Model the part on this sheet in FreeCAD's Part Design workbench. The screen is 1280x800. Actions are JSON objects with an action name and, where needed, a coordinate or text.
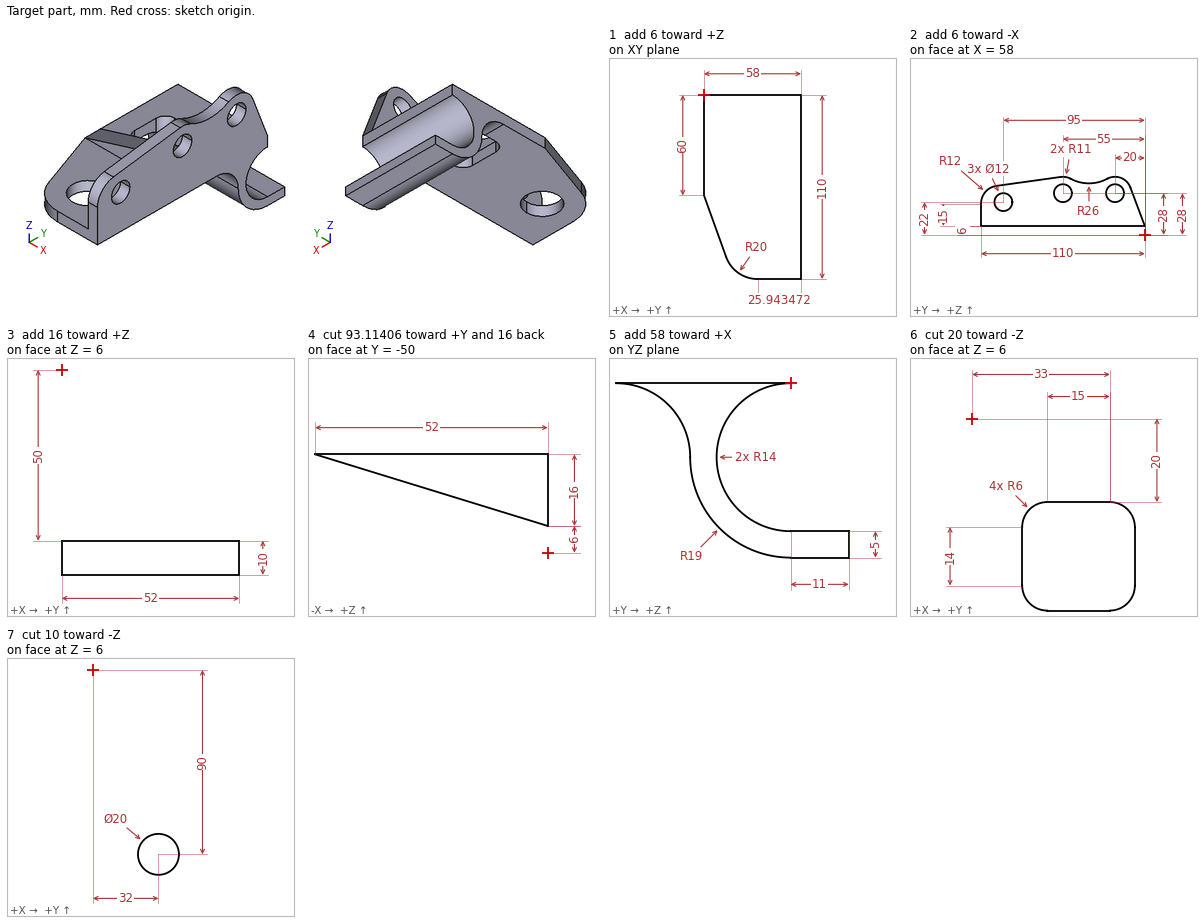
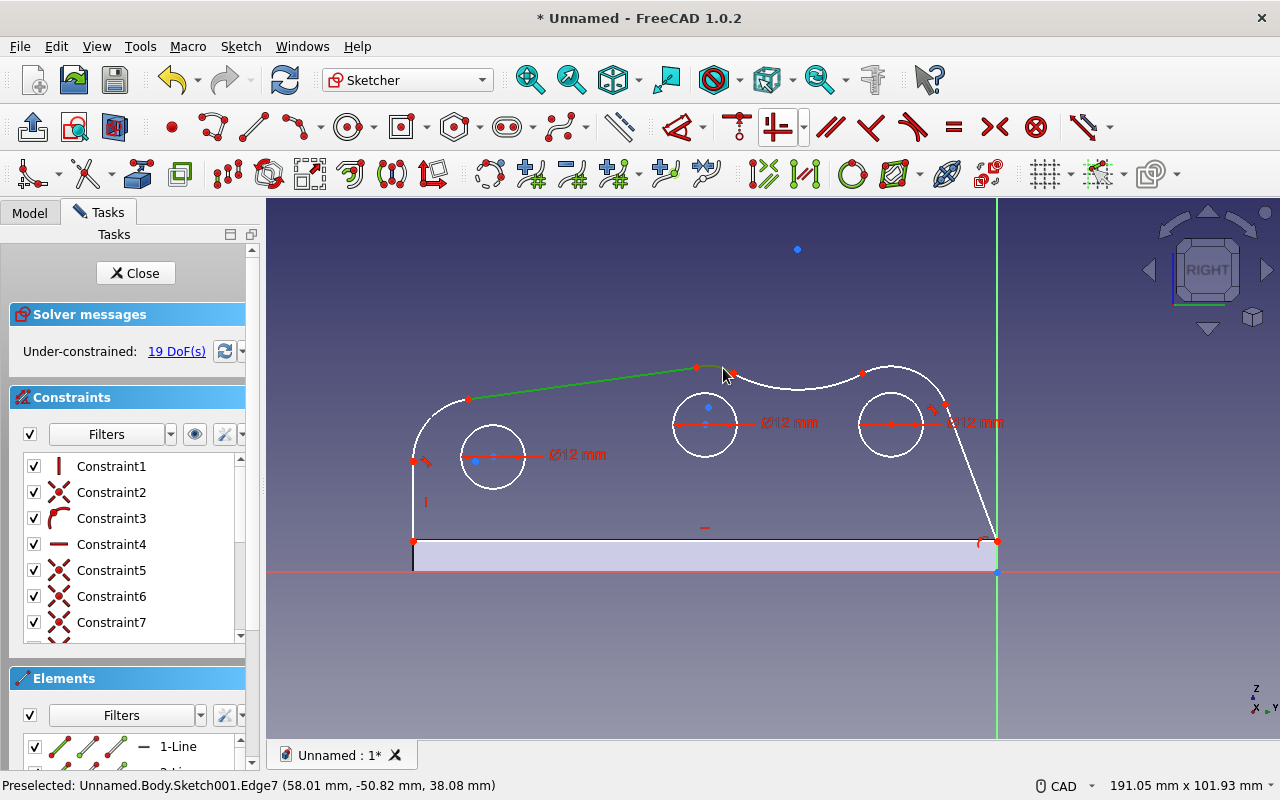
{"action": "key", "text": "t"}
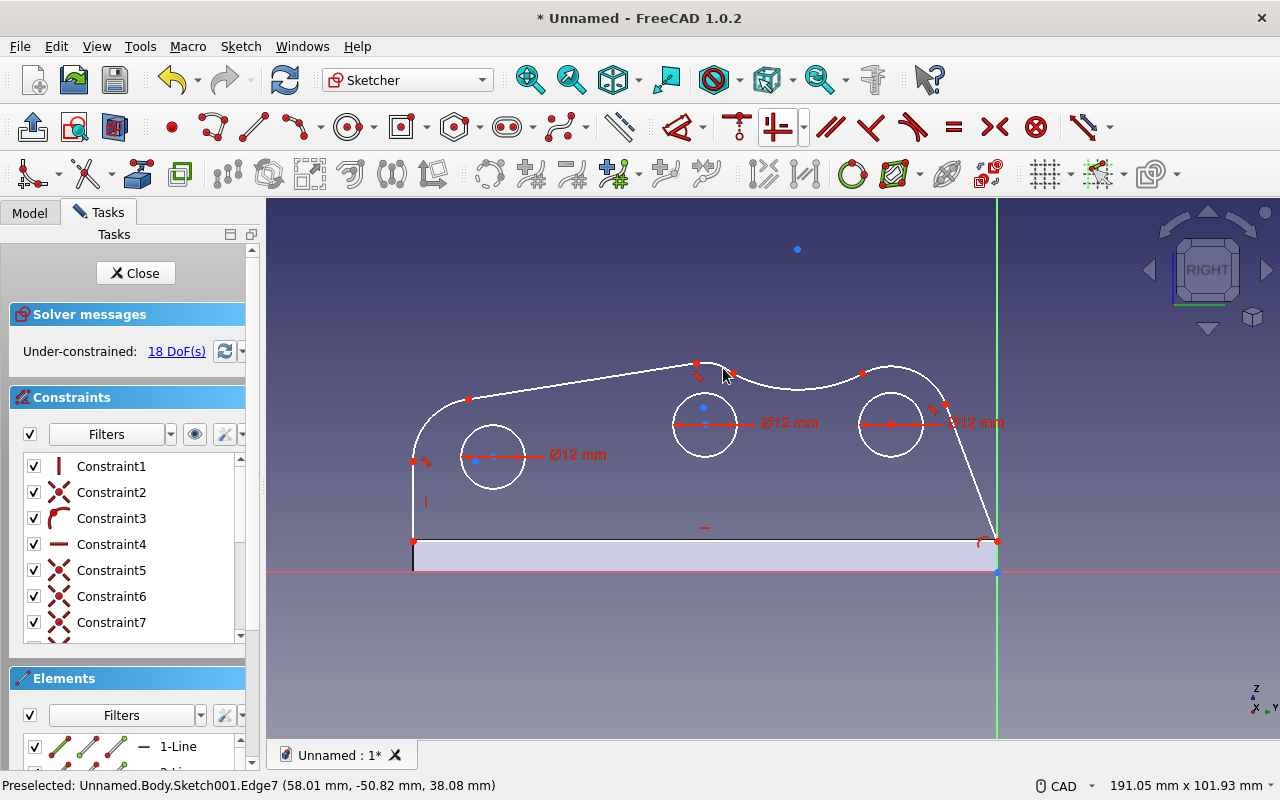
{"action": "left_click", "coordinate": [628, 374]}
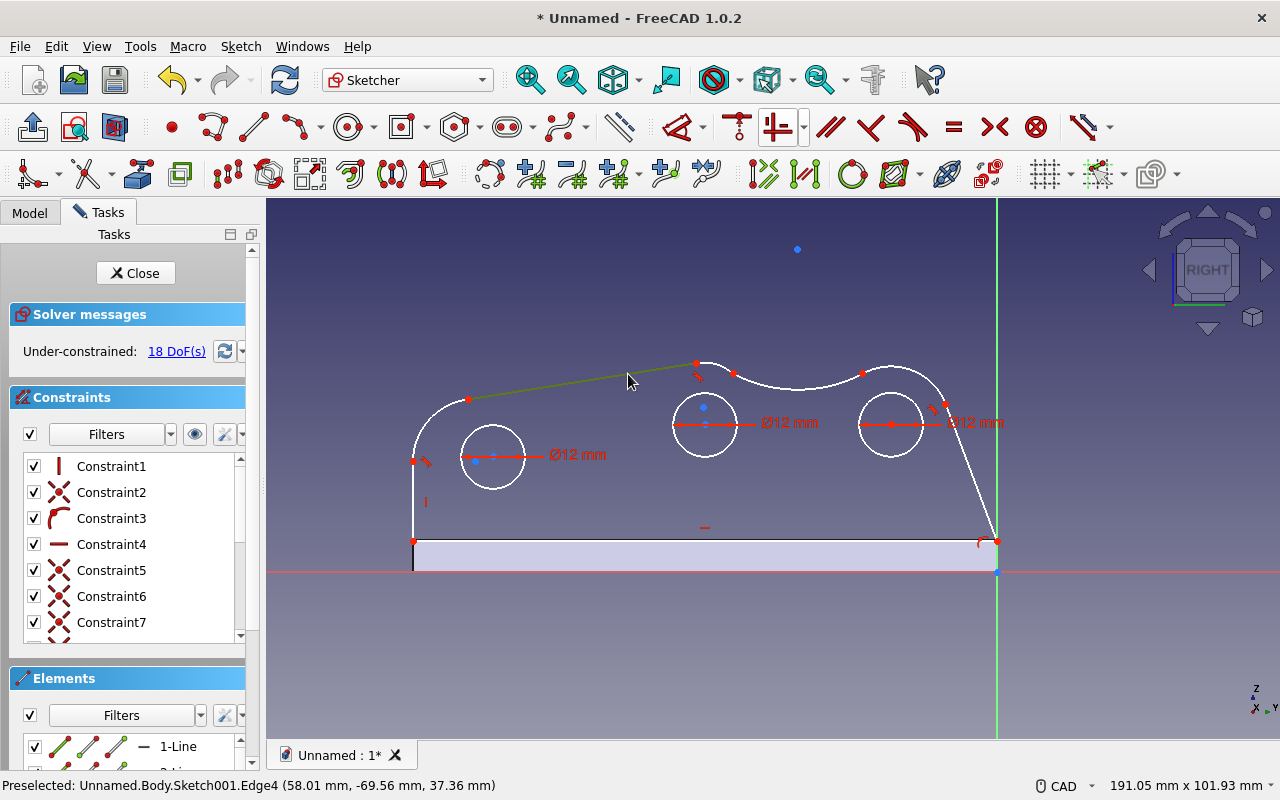
{"action": "left_click", "coordinate": [443, 408]}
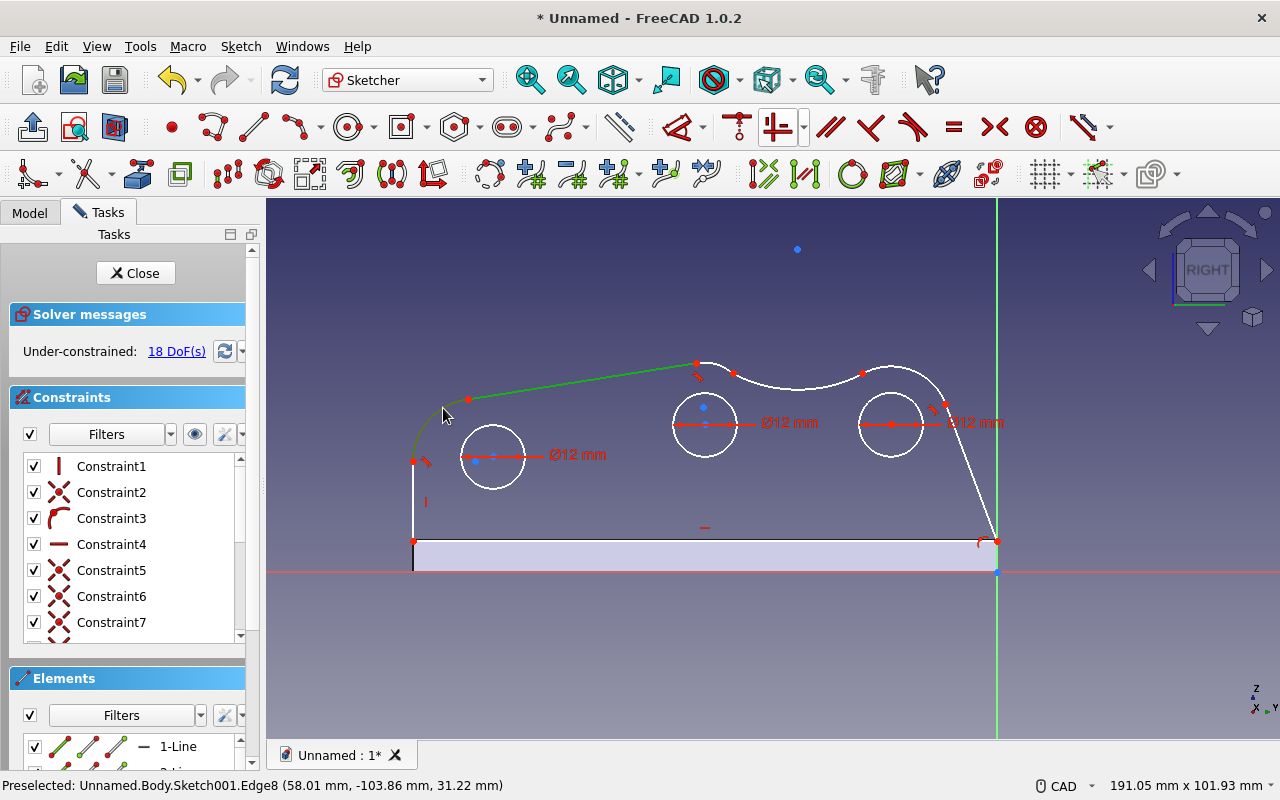
{"action": "left_click", "coordinate": [913, 128]}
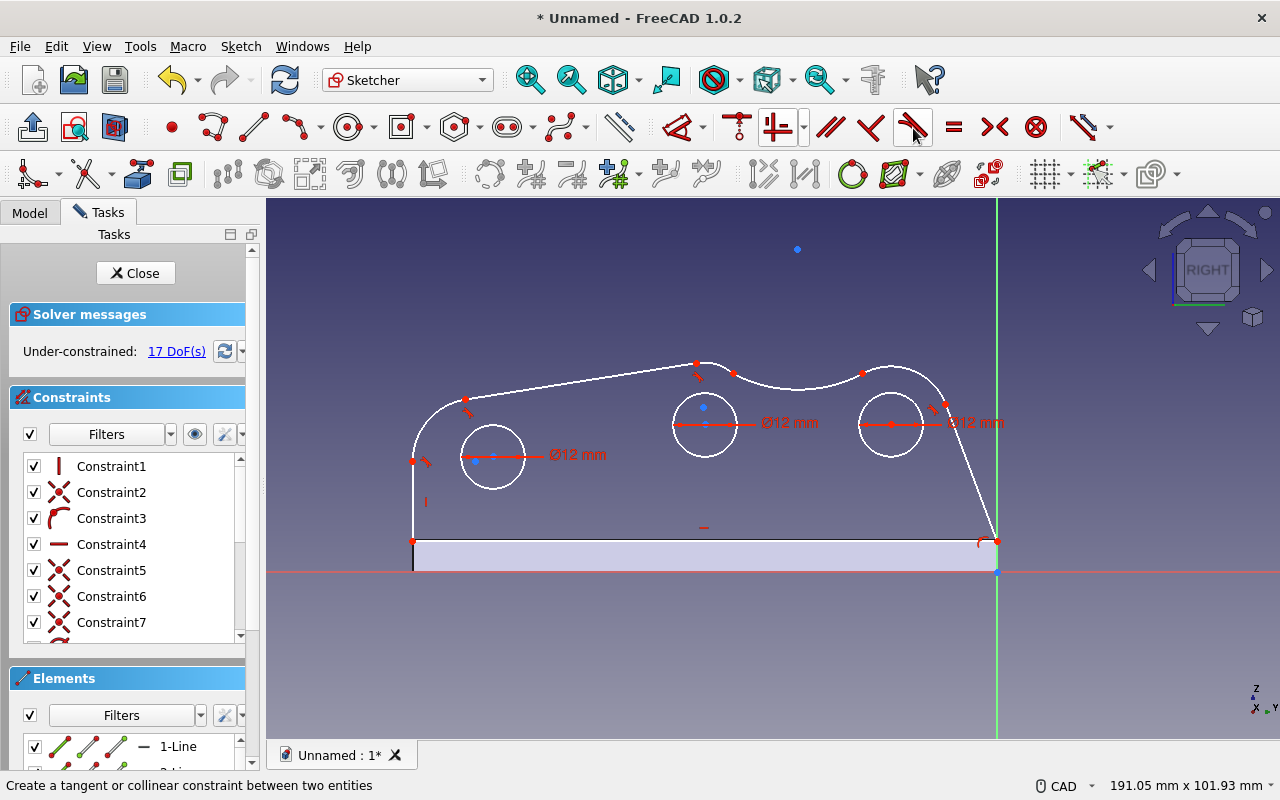
{"action": "left_click", "coordinate": [928, 380]}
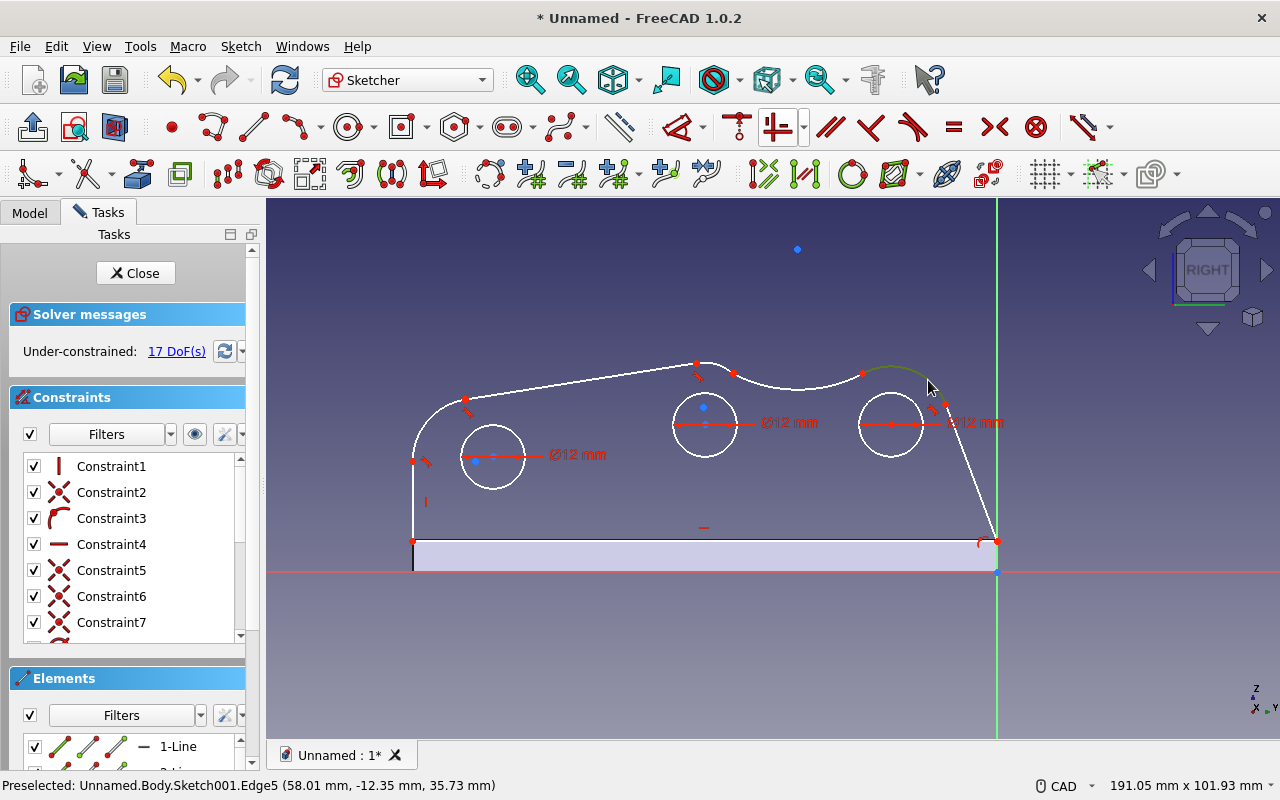
{"action": "left_click", "coordinate": [771, 387]}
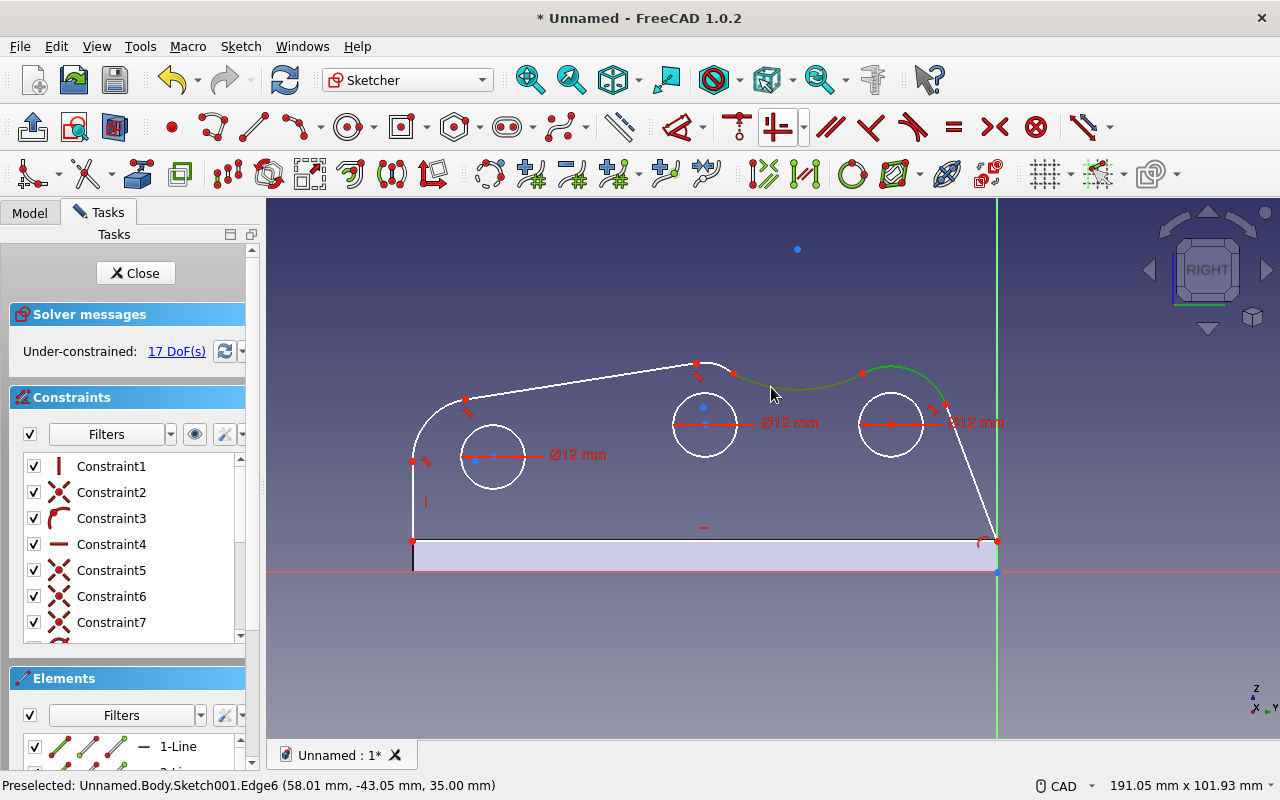
{"action": "left_click", "coordinate": [913, 128]}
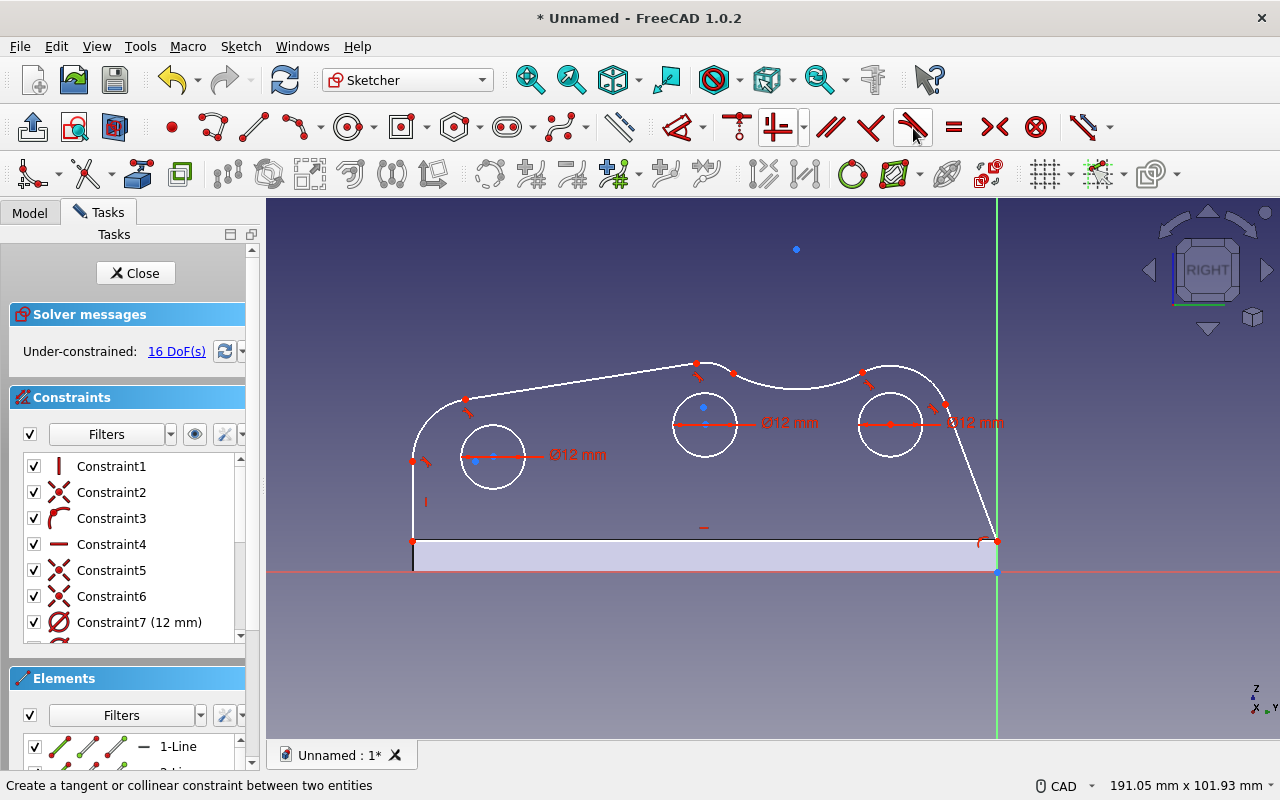
{"action": "left_click", "coordinate": [771, 387]}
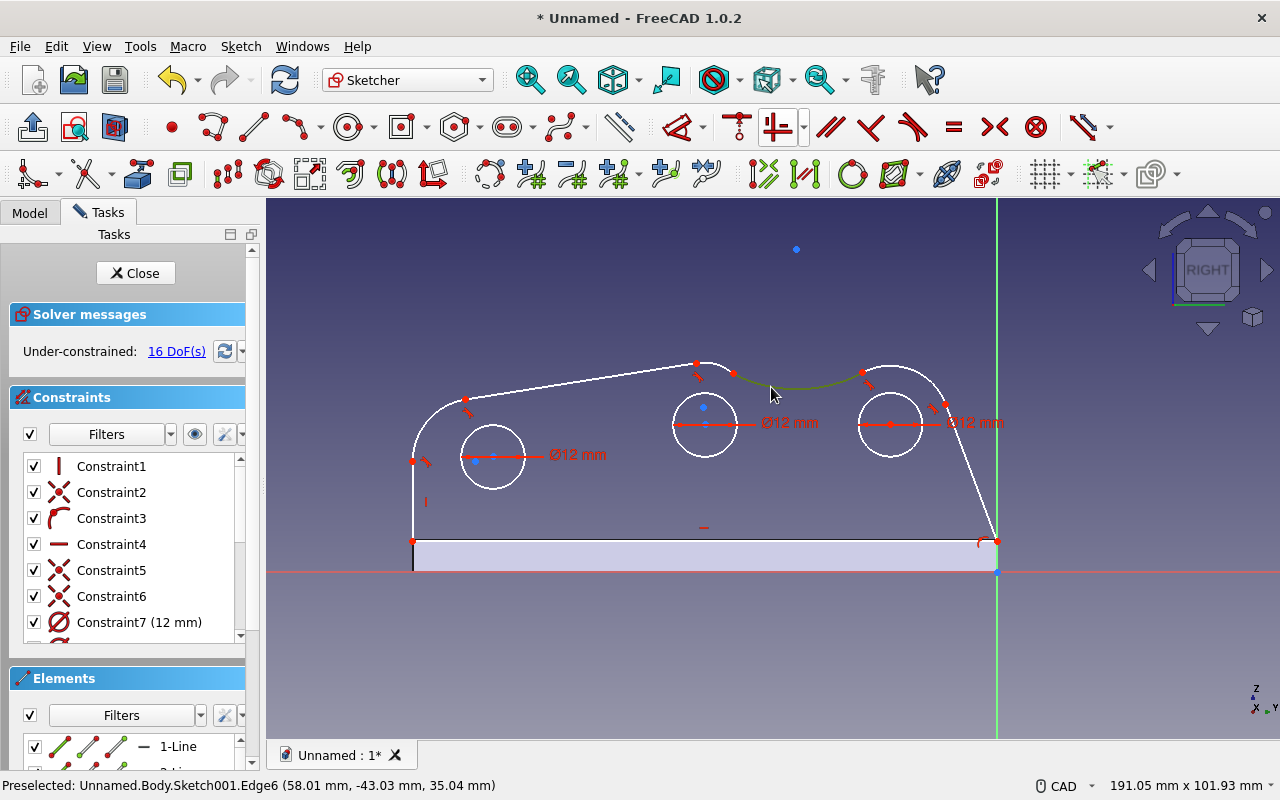
{"action": "left_click", "coordinate": [723, 367]}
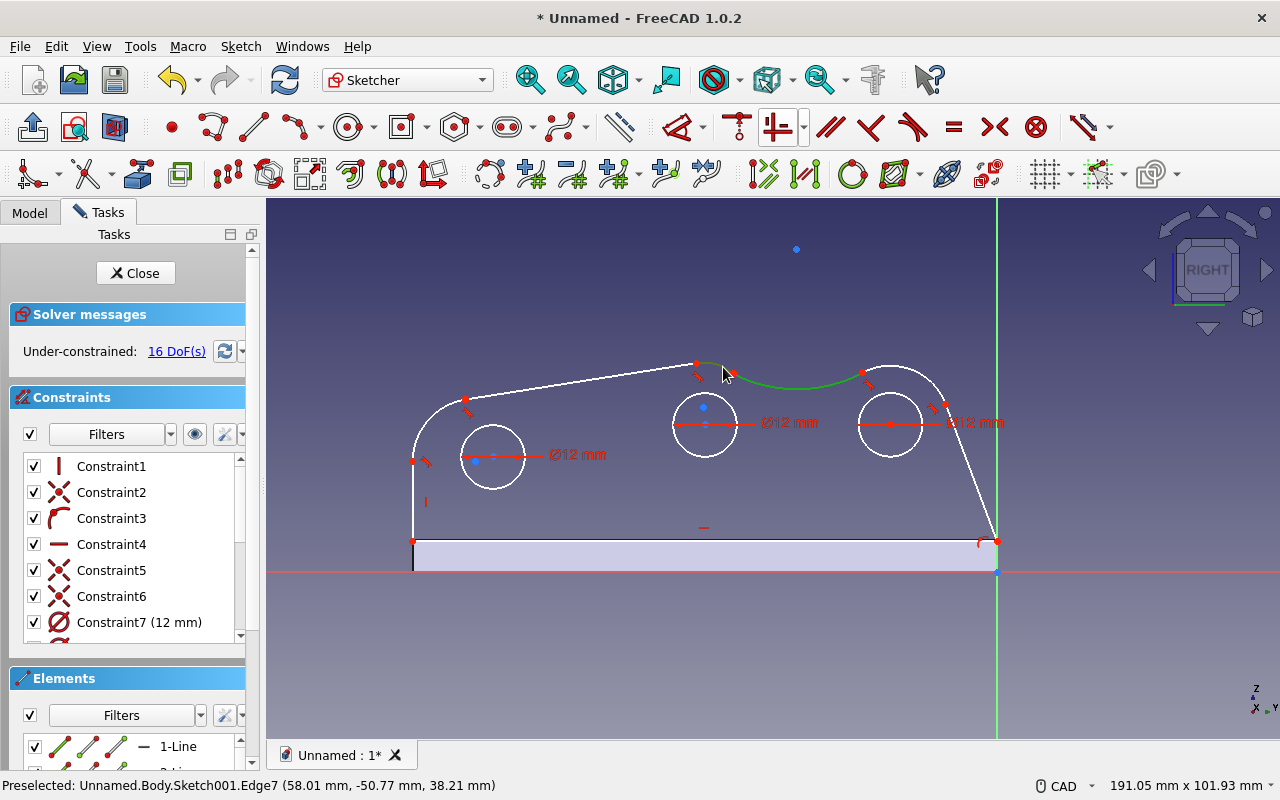
{"action": "left_click", "coordinate": [913, 128]}